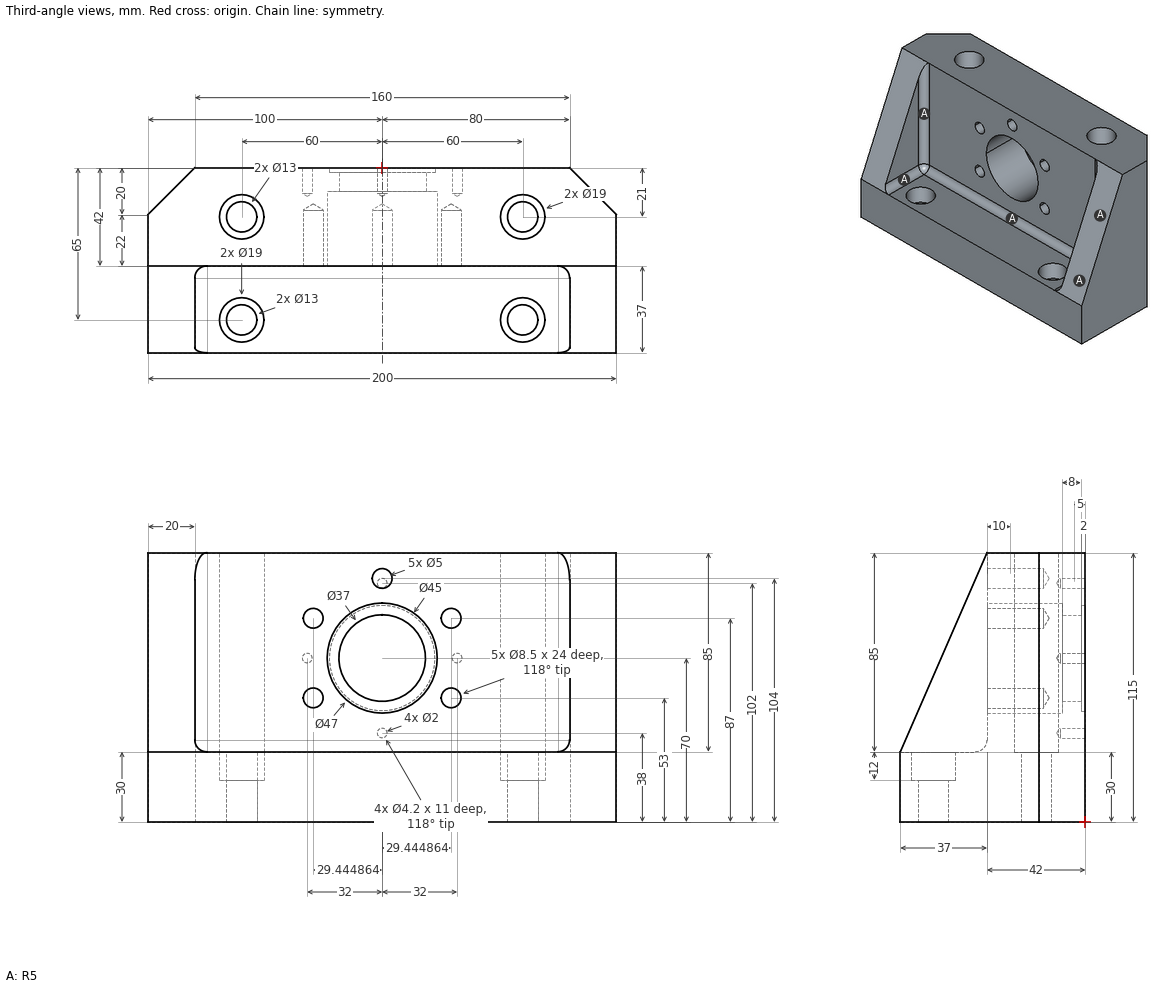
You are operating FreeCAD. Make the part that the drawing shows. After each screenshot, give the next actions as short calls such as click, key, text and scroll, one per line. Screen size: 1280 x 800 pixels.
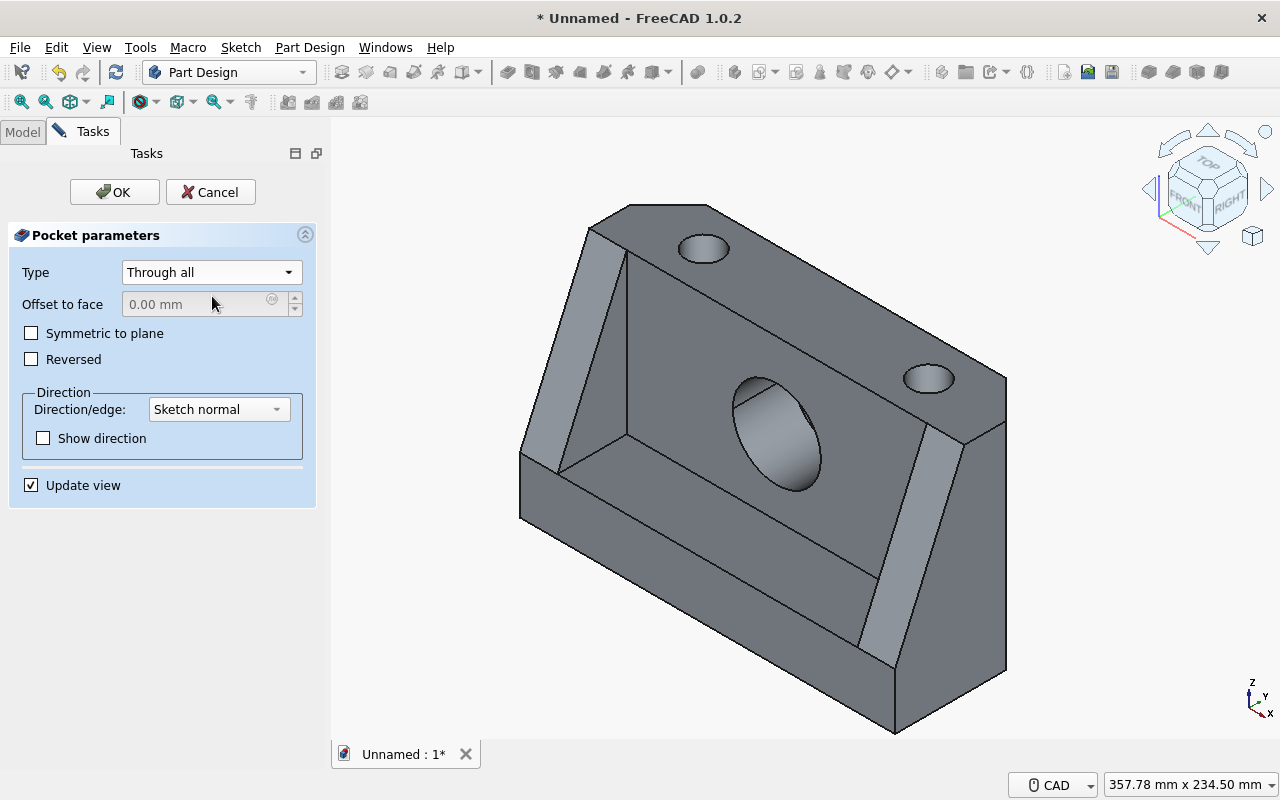
click(115, 192)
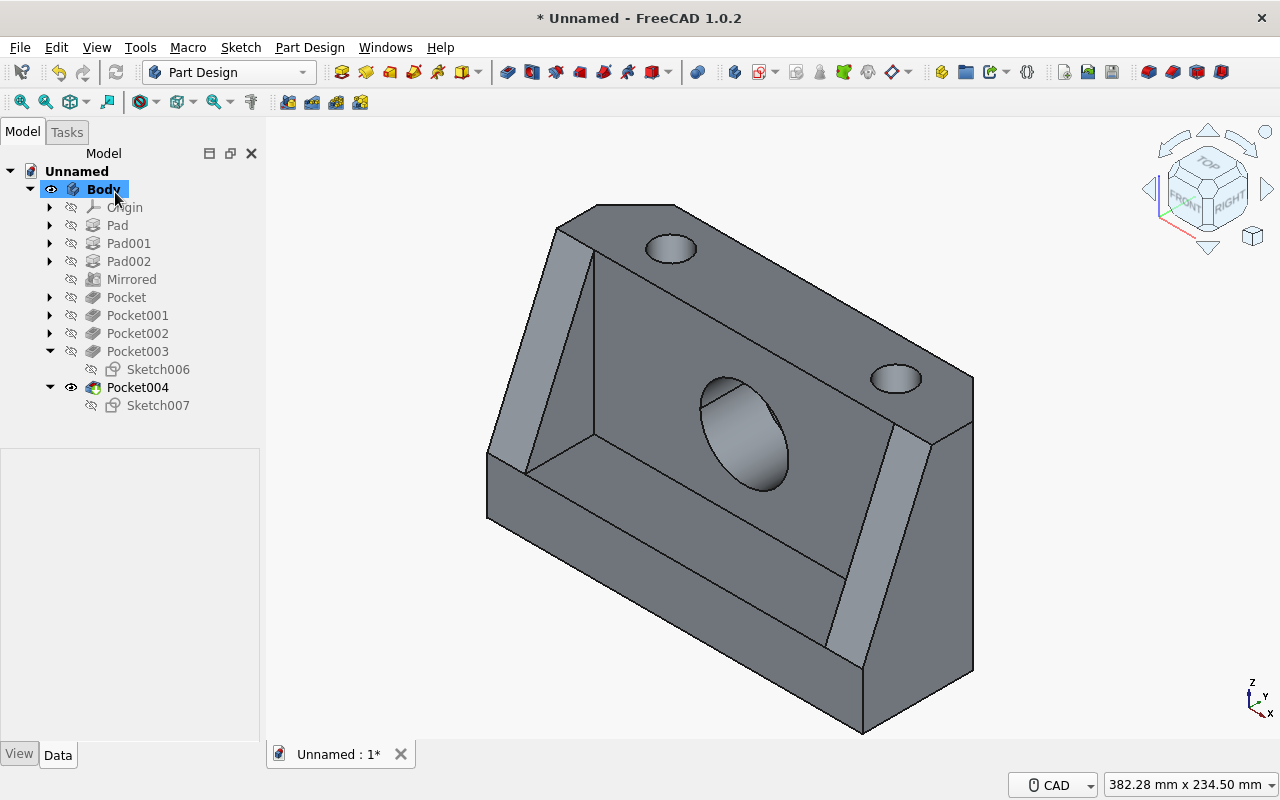
click(830, 451)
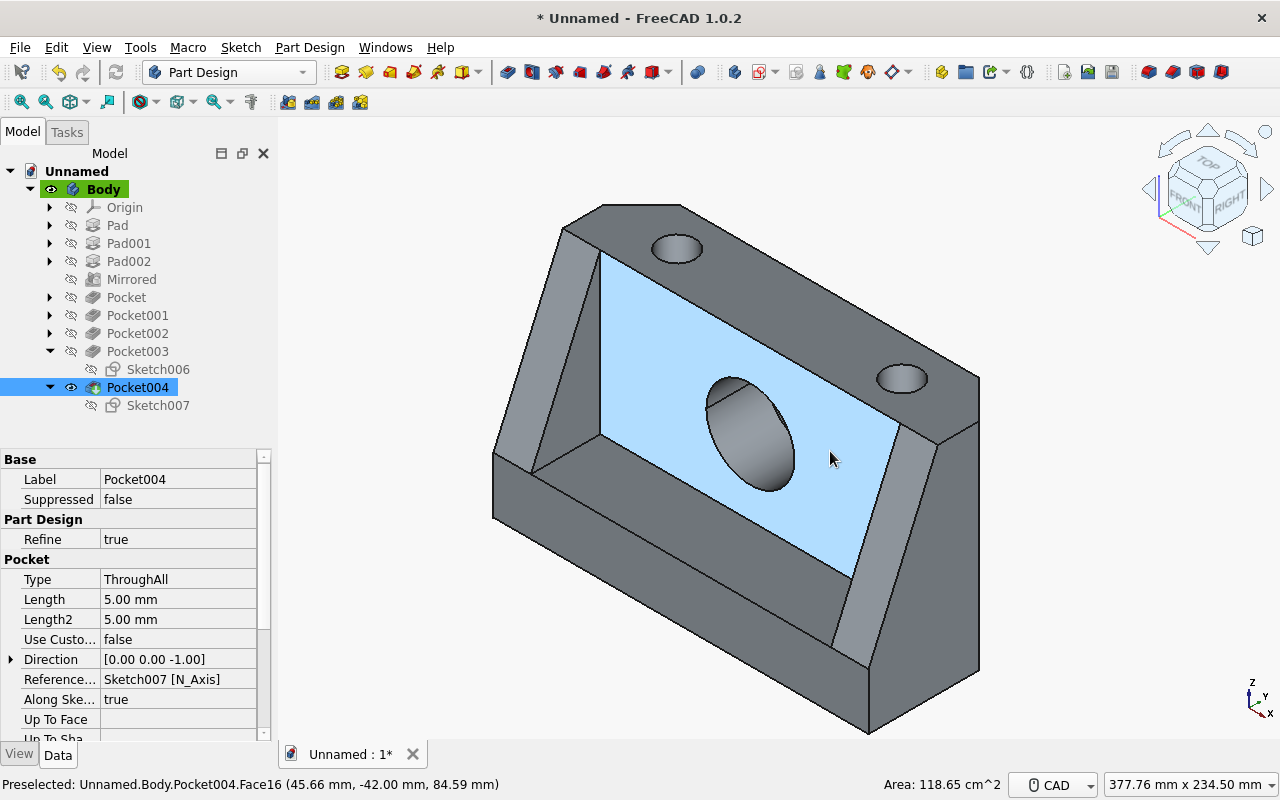
click(760, 72)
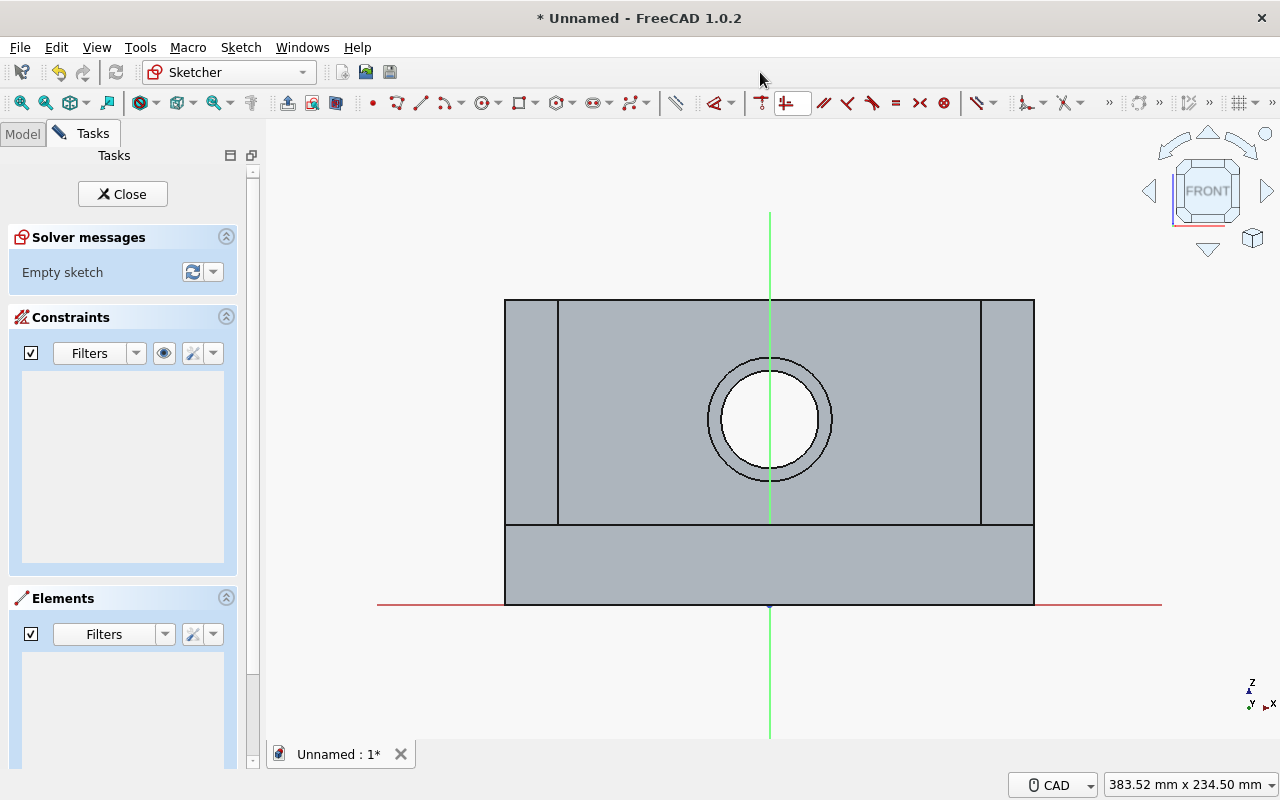
click(336, 104)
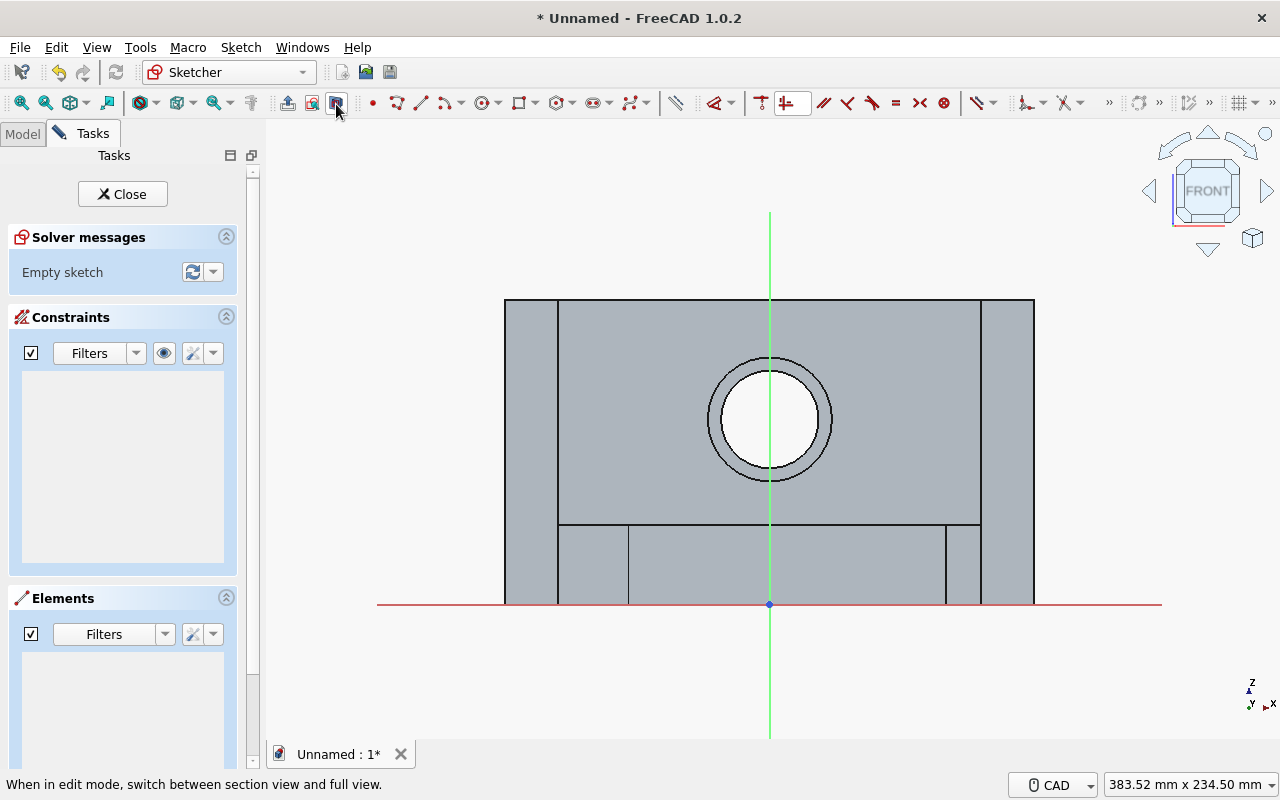
scroll(903, 534, up, 2)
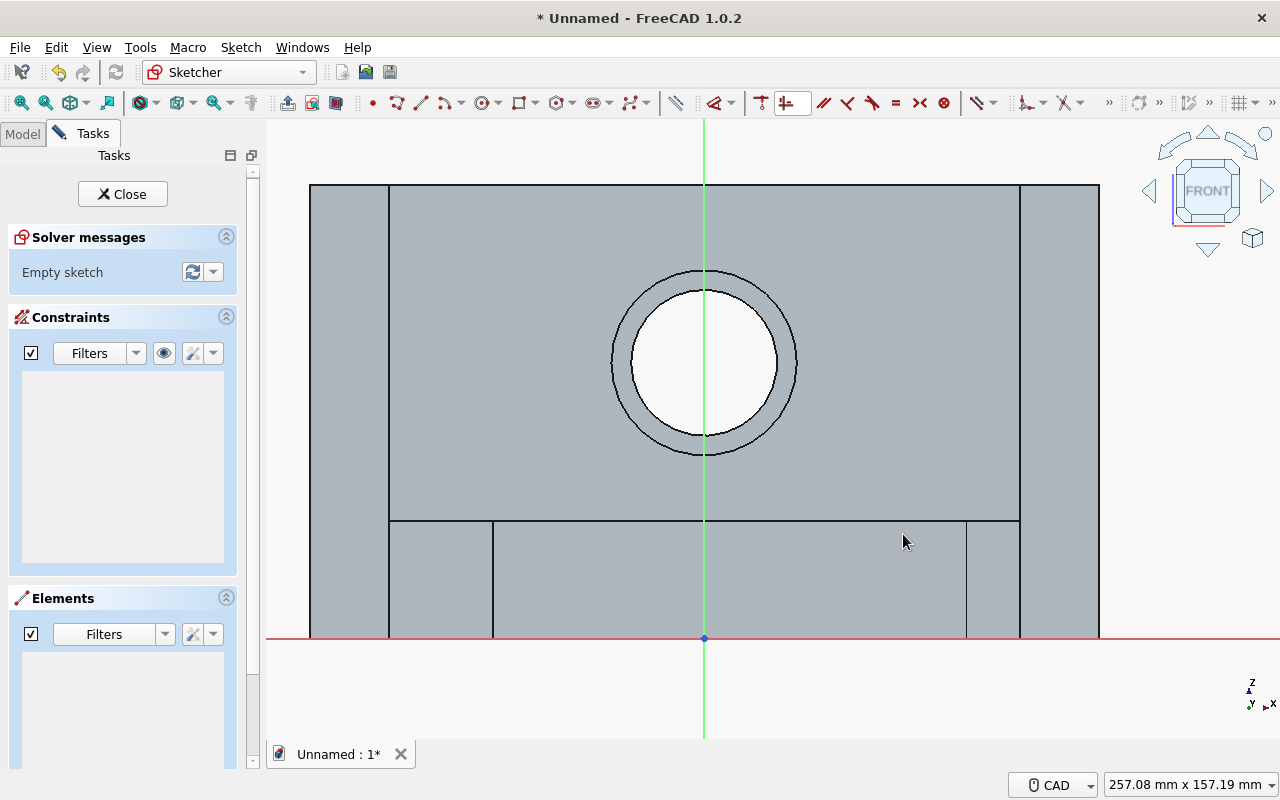
key(g)
key(c)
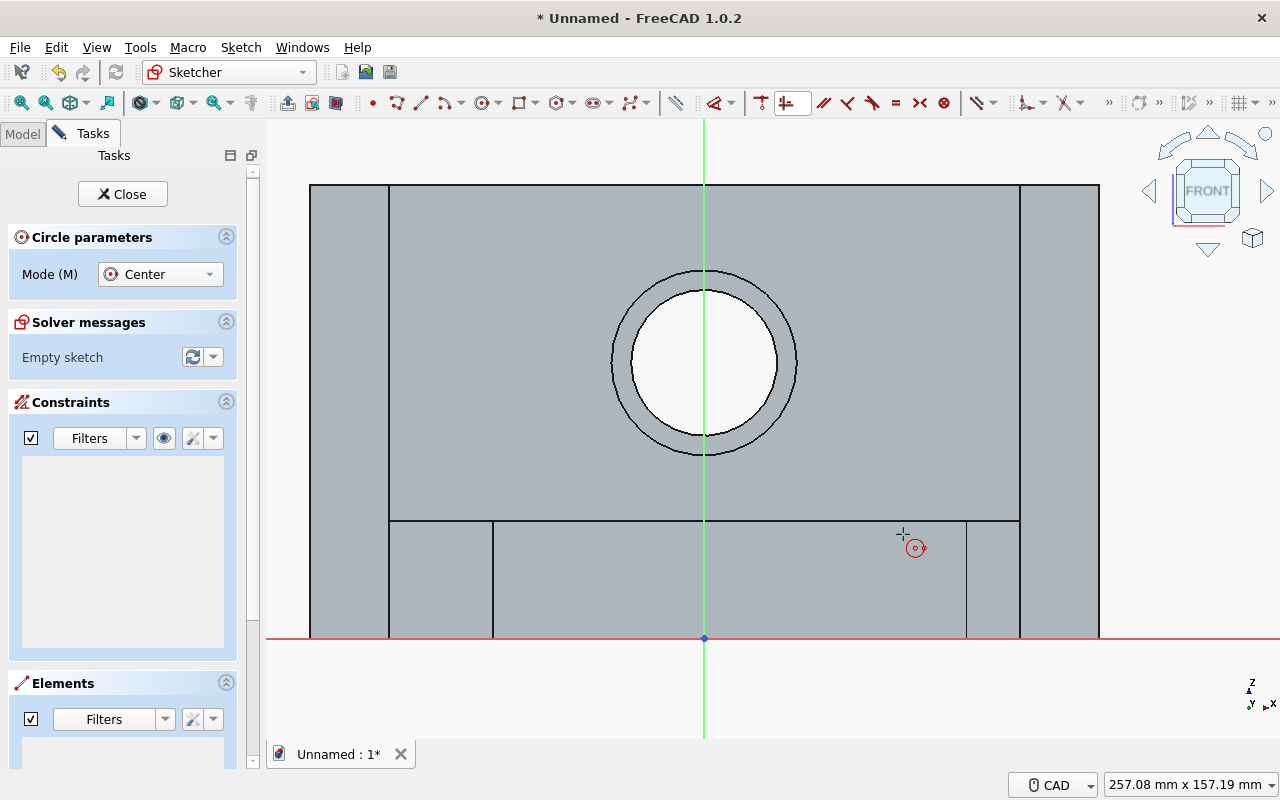
scroll(704, 229, up, 5)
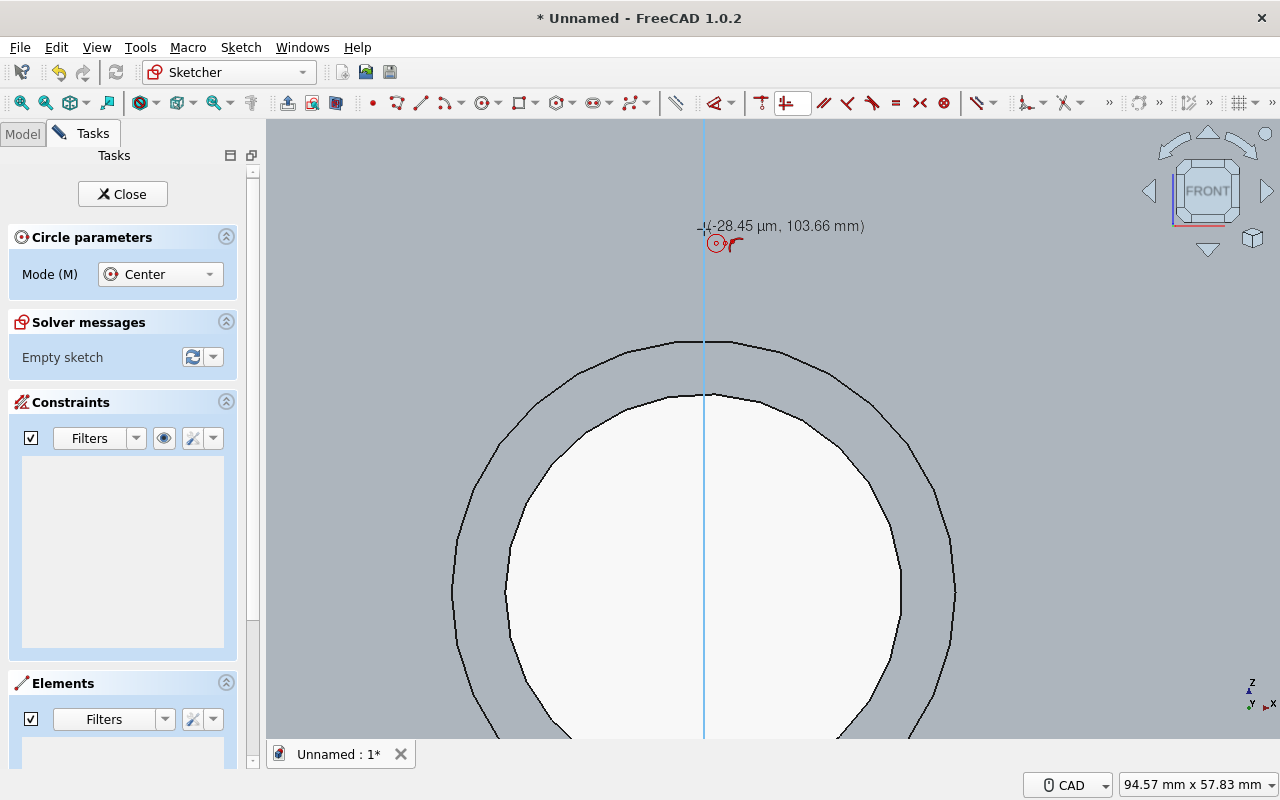
click(704, 228)
move(723, 209)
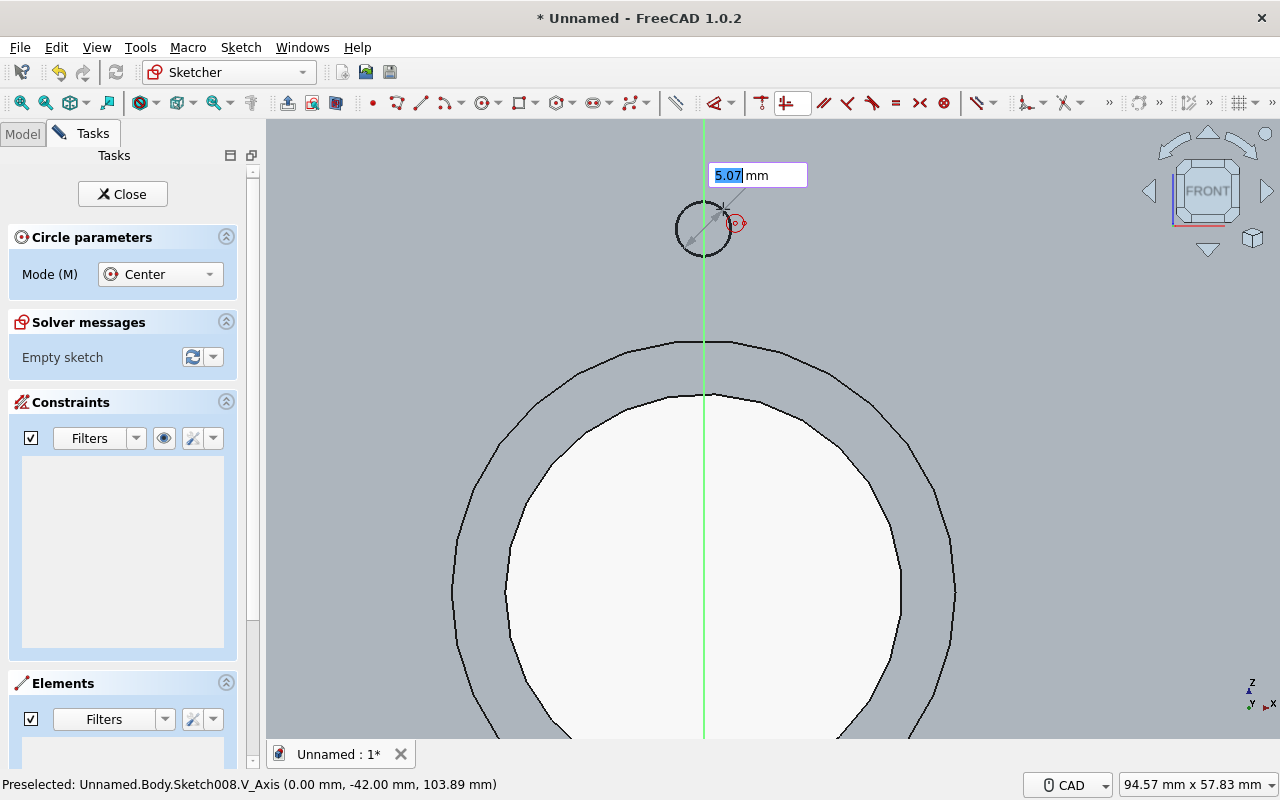
text(5)
key(Return)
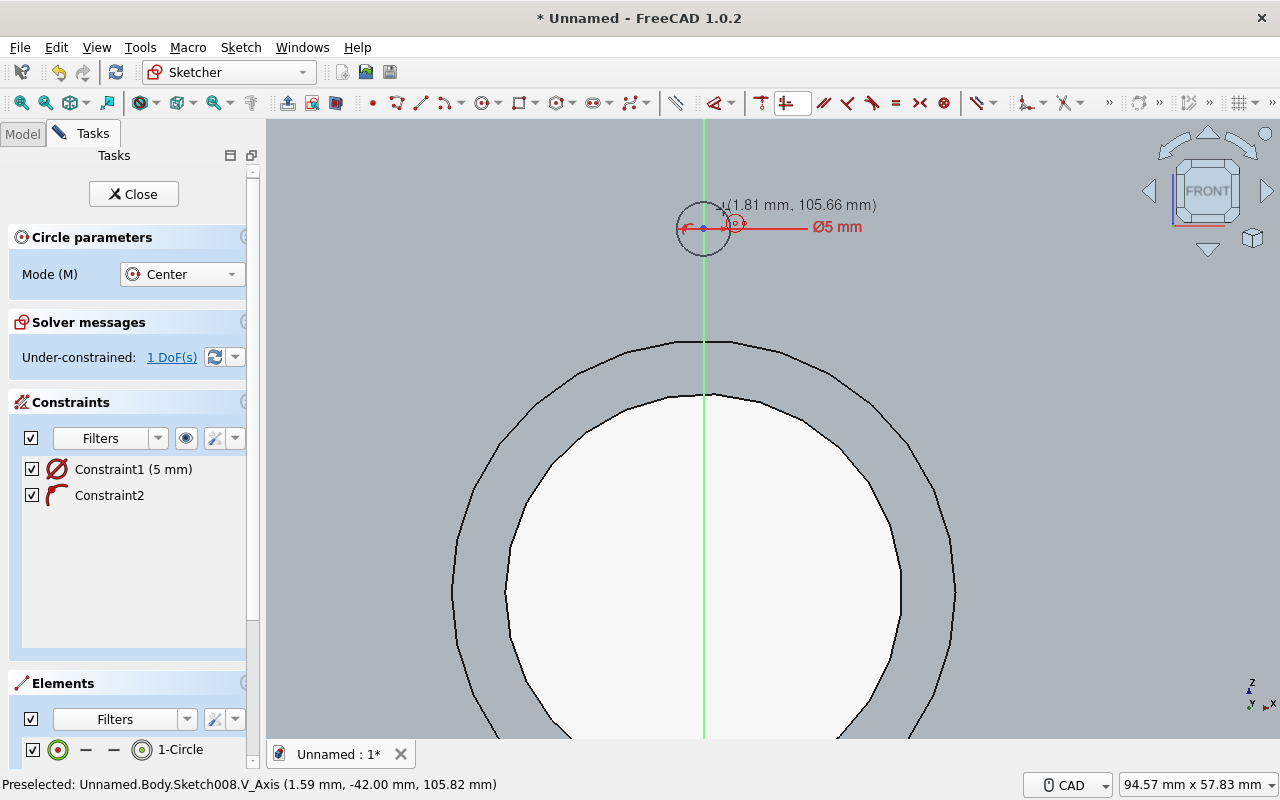
click(1019, 410)
move(1038, 391)